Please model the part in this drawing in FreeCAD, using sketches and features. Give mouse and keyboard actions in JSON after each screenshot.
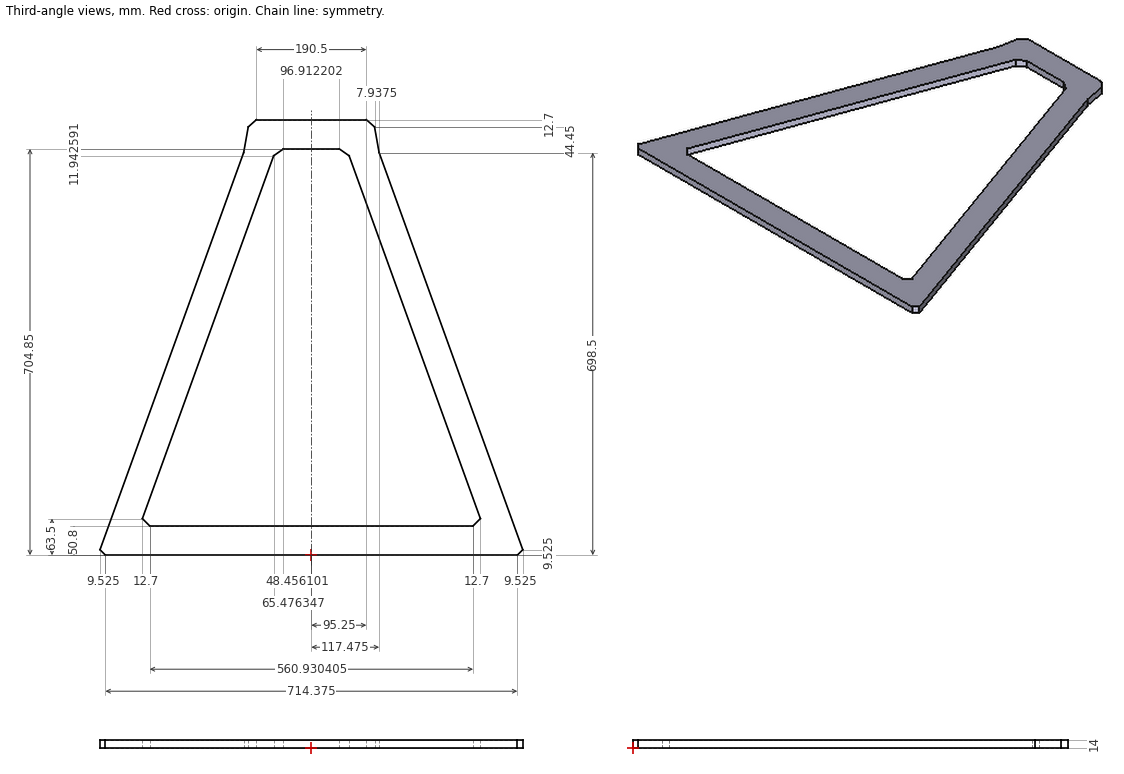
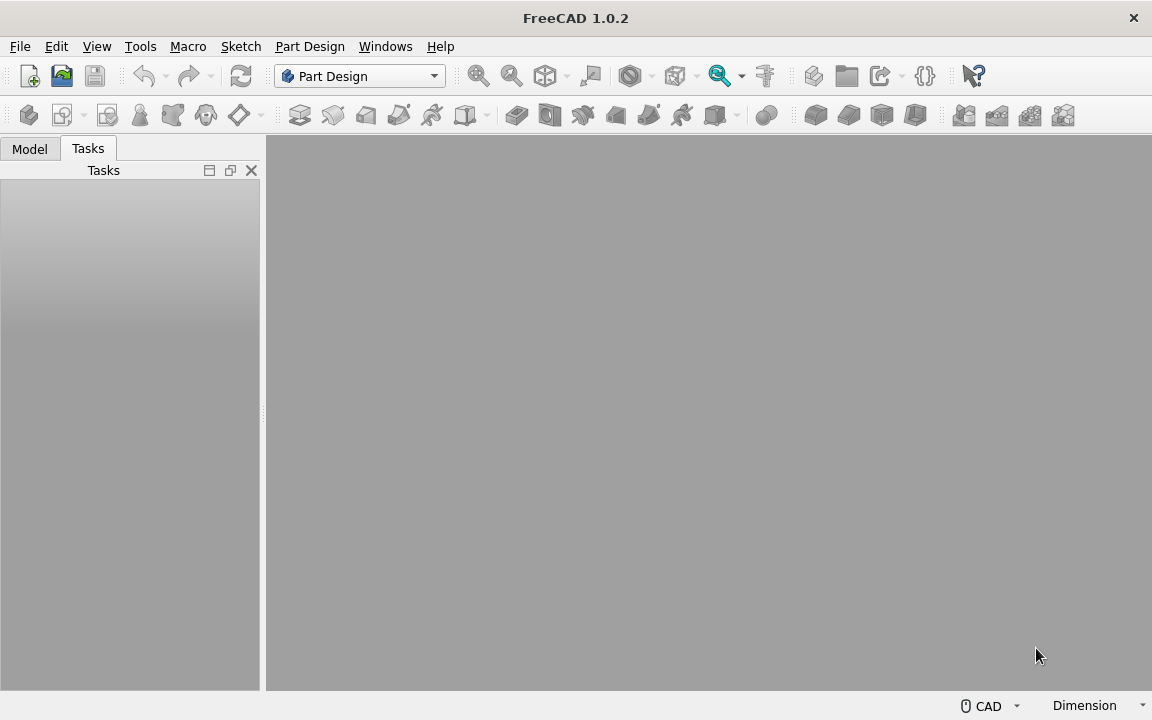
{"action": "left_click", "coordinate": [29, 76]}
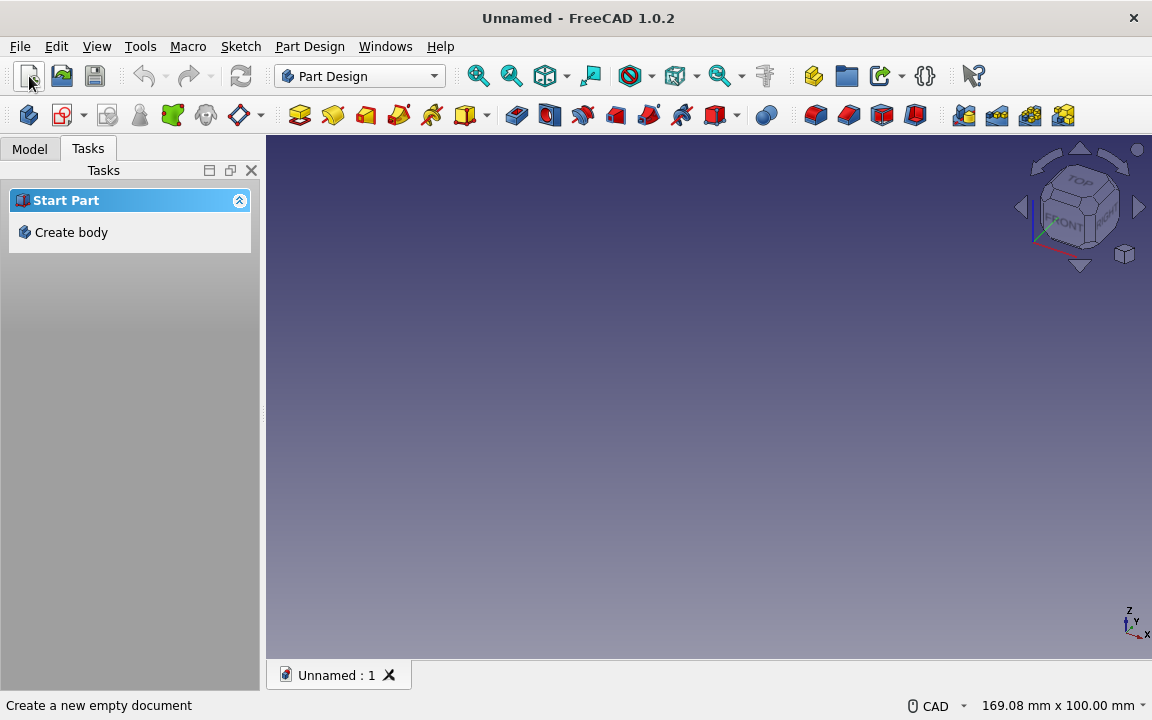
{"action": "left_click", "coordinate": [62, 116]}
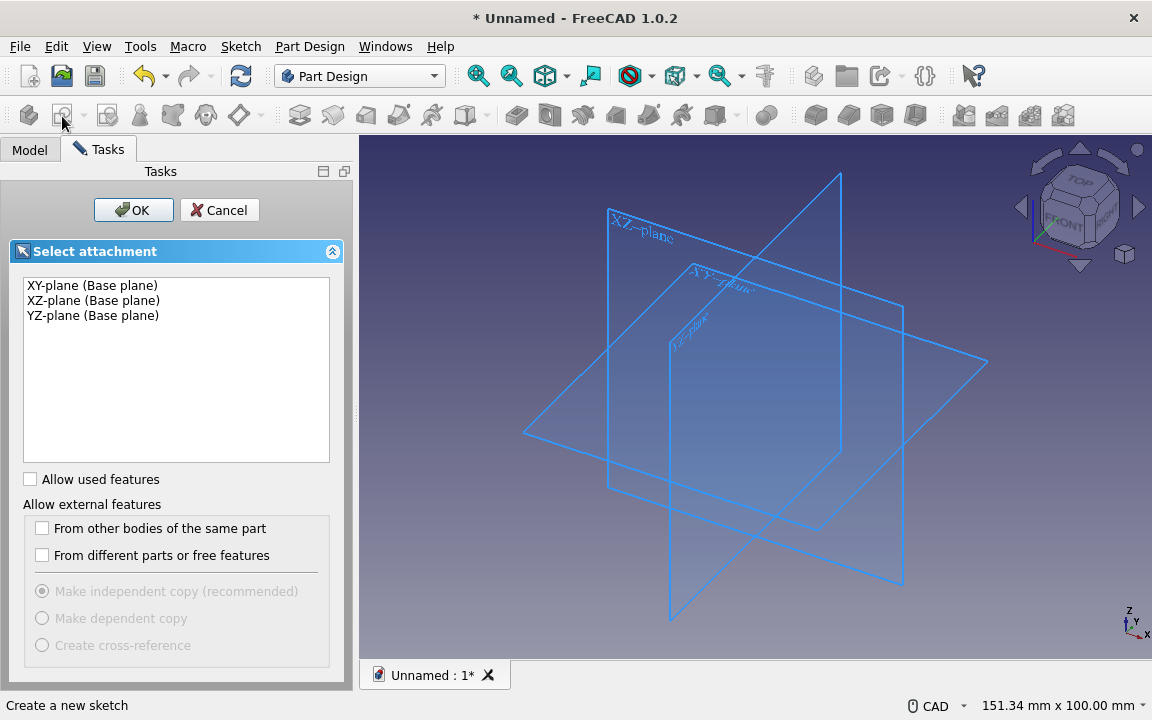
{"action": "left_click", "coordinate": [84, 286]}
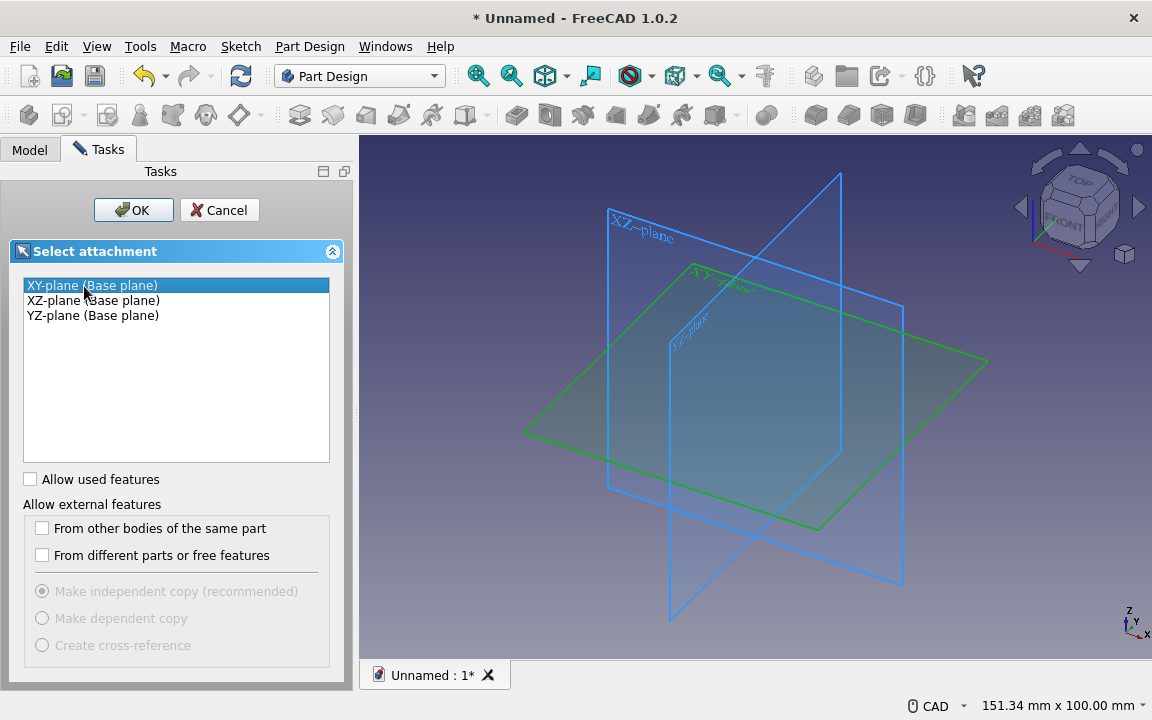
{"action": "left_click", "coordinate": [134, 210]}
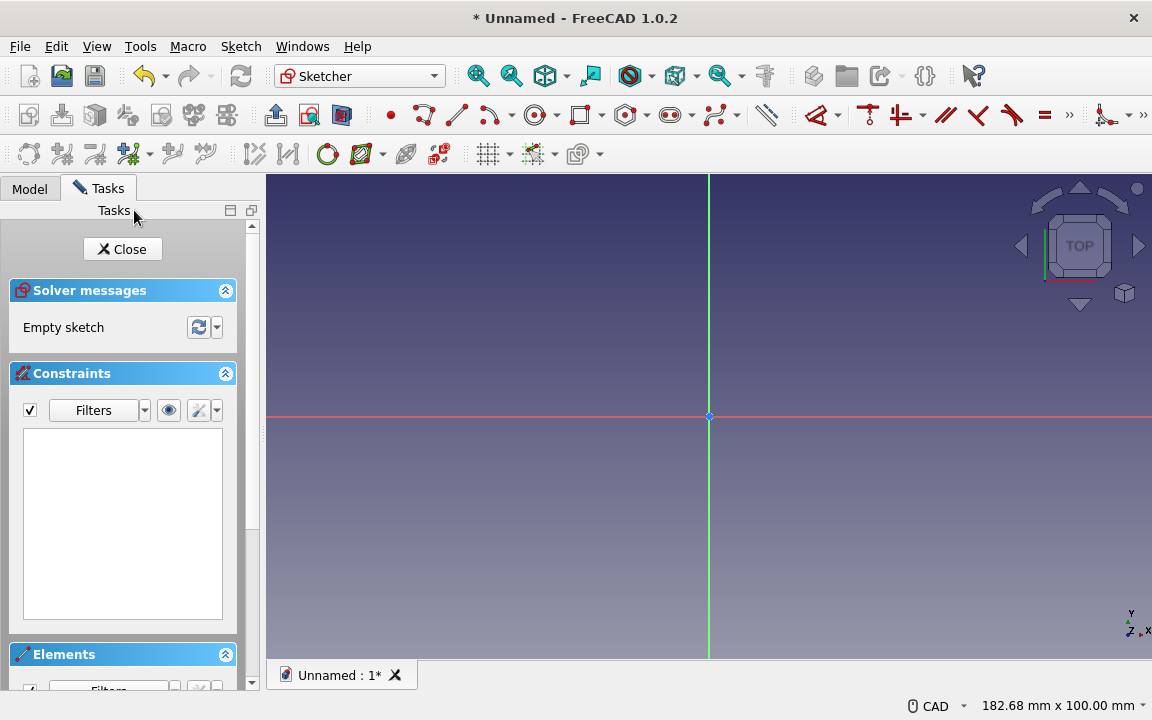
{"action": "scroll", "coordinate": [634, 599], "scroll_direction": "down", "scroll_amount": 12}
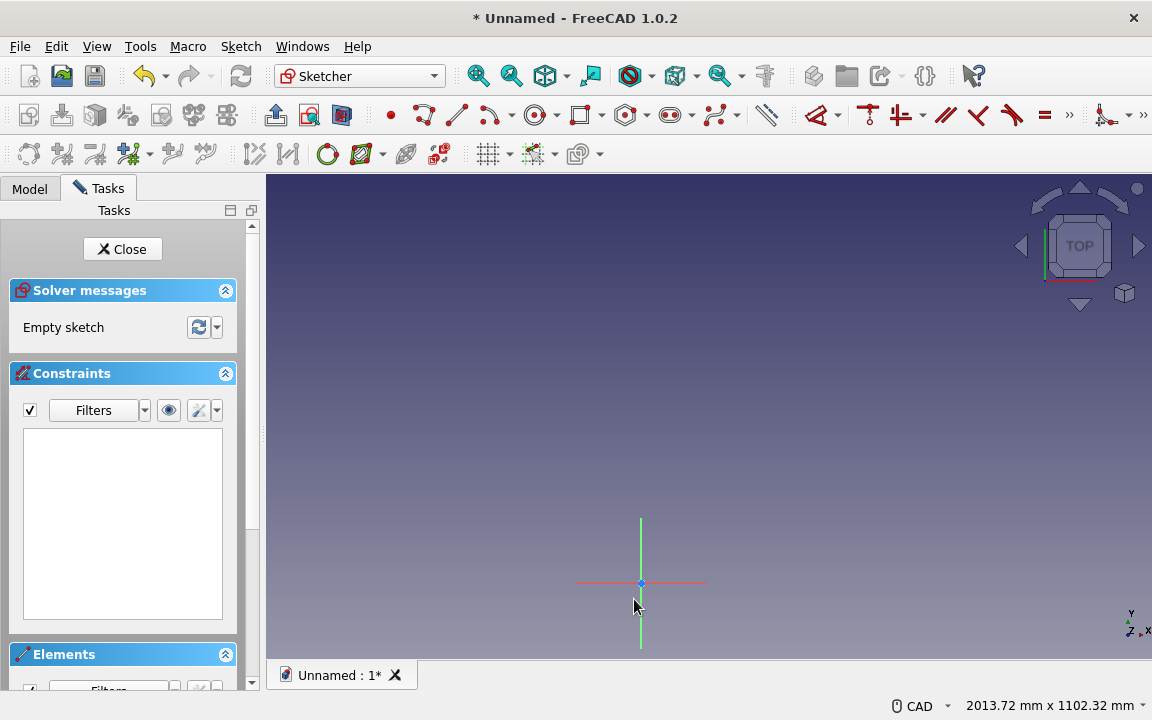
{"action": "left_click", "coordinate": [424, 116]}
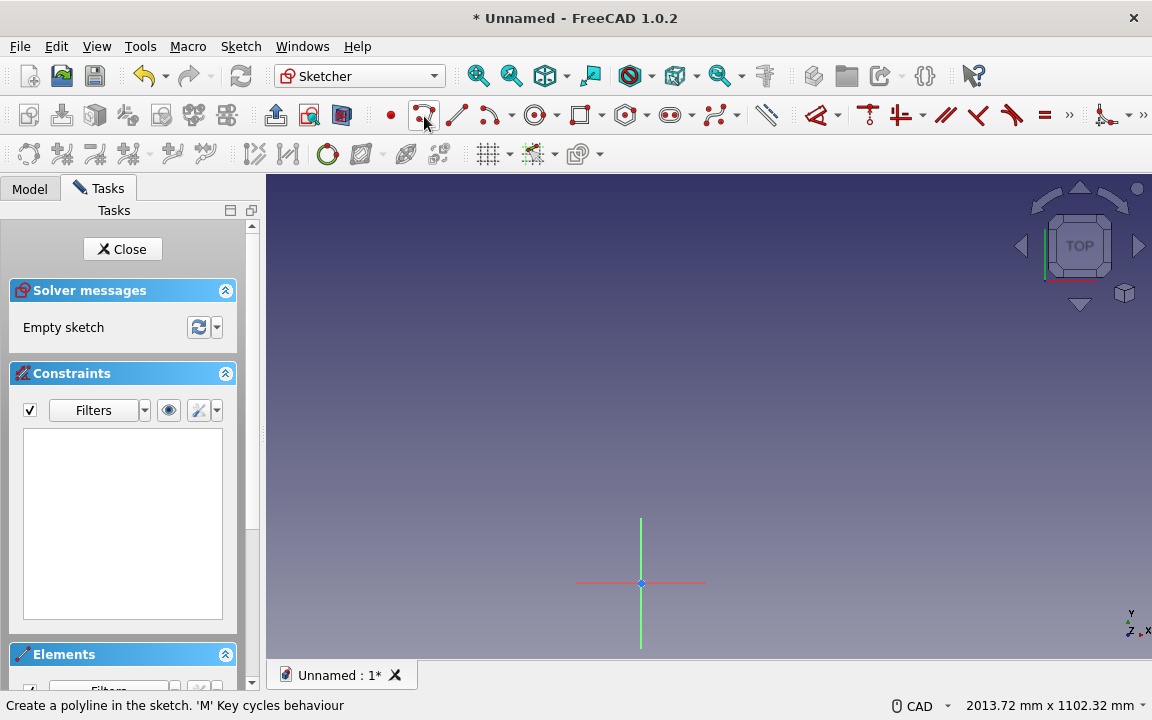
{"action": "left_click", "coordinate": [484, 583]}
{"action": "left_click", "coordinate": [798, 574]}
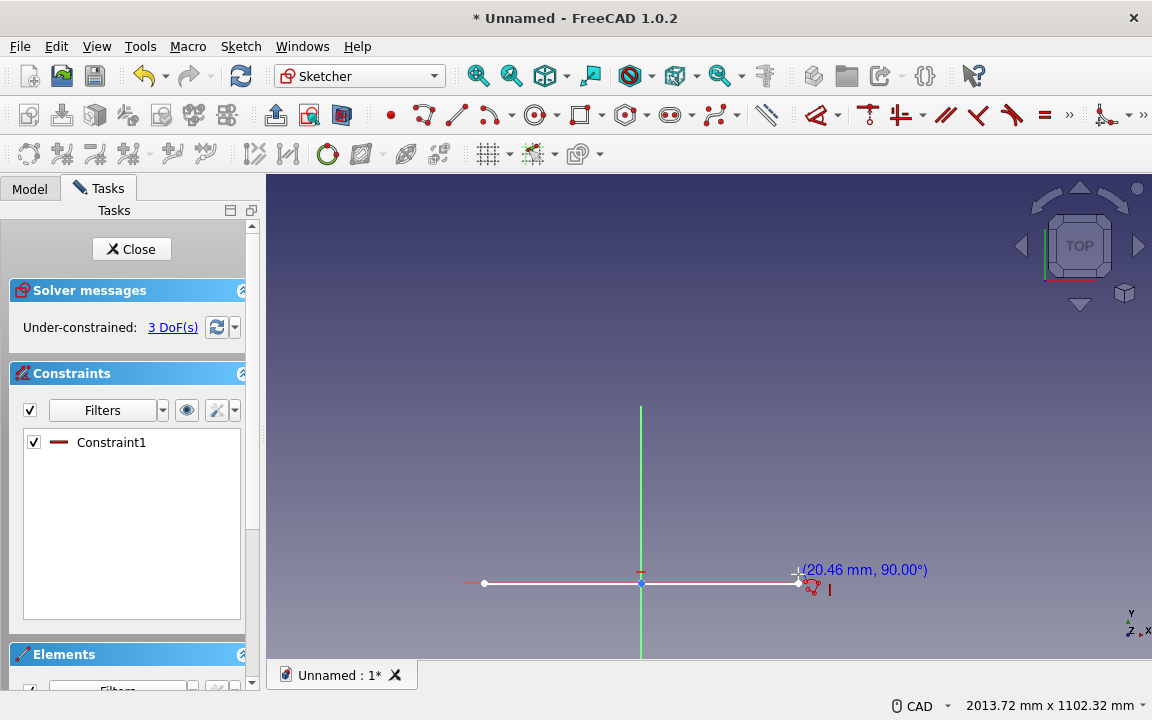
{"action": "scroll", "coordinate": [803, 579], "scroll_direction": "up", "scroll_amount": 7}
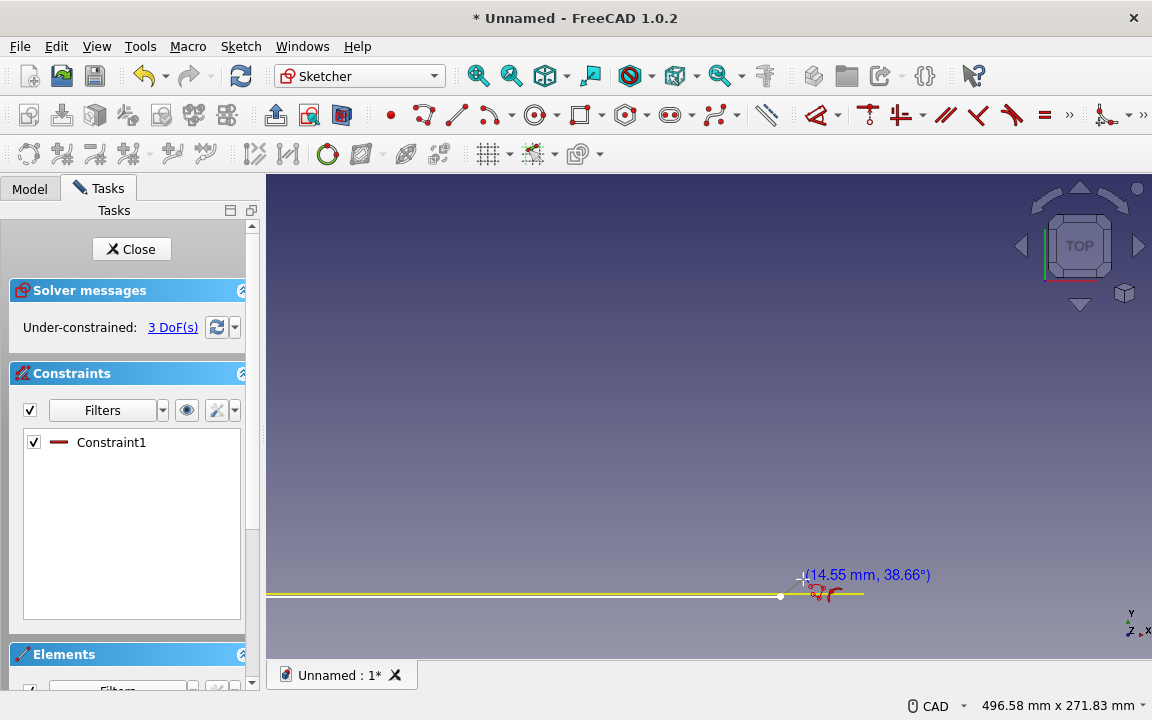
{"action": "left_click", "coordinate": [799, 577]}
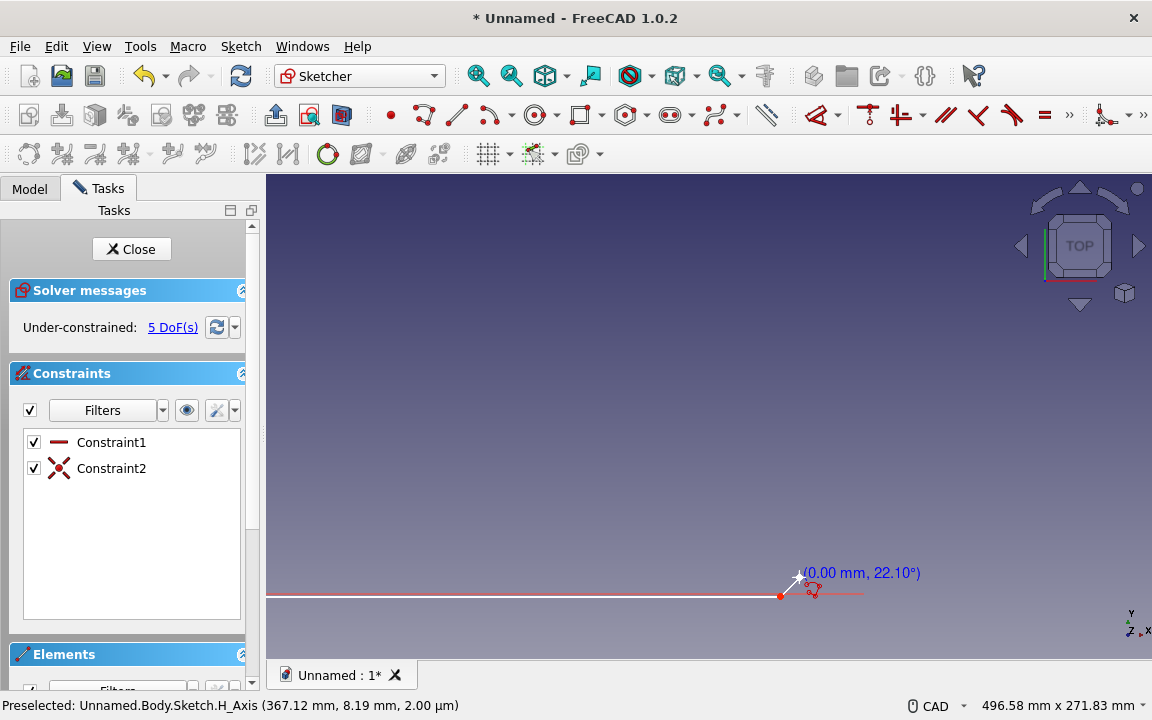
{"action": "scroll", "coordinate": [803, 579], "scroll_direction": "down", "scroll_amount": 7}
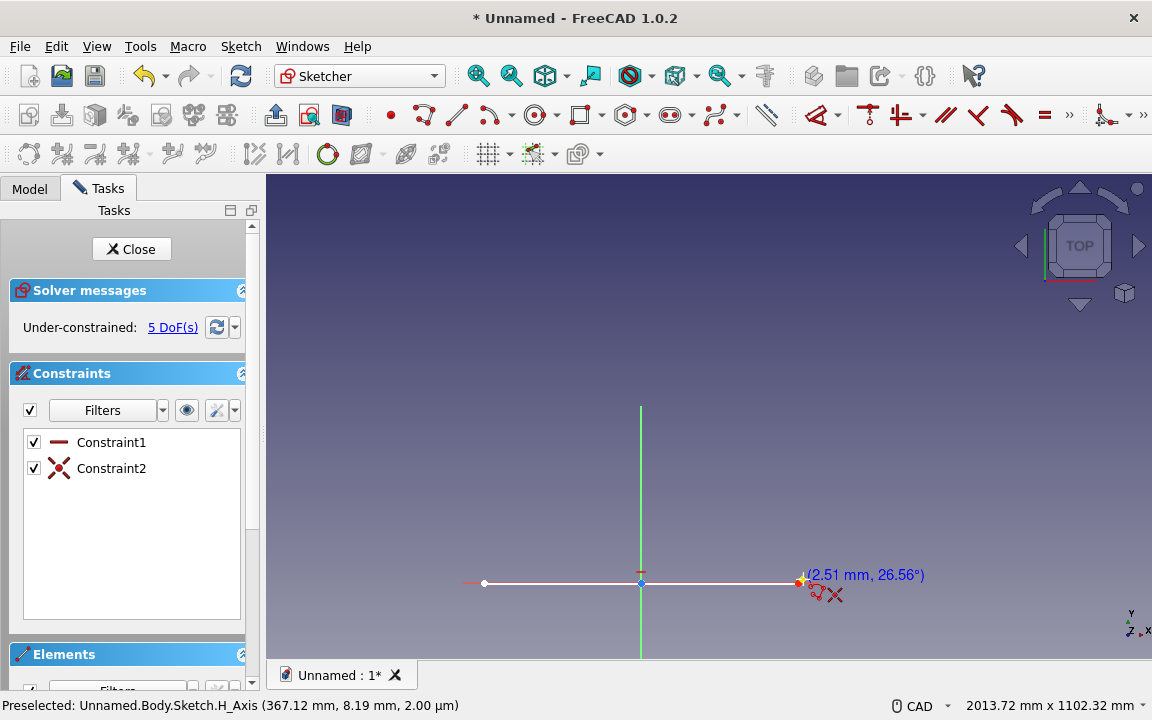
{"action": "left_click", "coordinate": [693, 276]}
{"action": "left_click", "coordinate": [689, 256]}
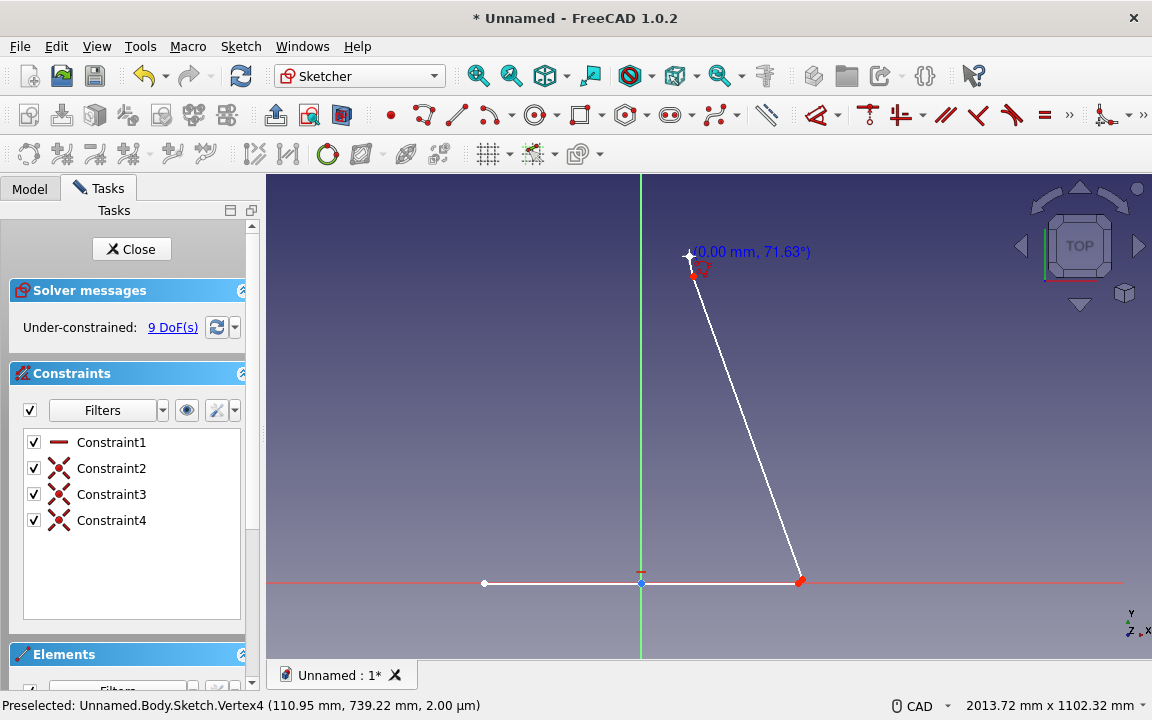
{"action": "scroll", "coordinate": [683, 251], "scroll_direction": "up", "scroll_amount": 4}